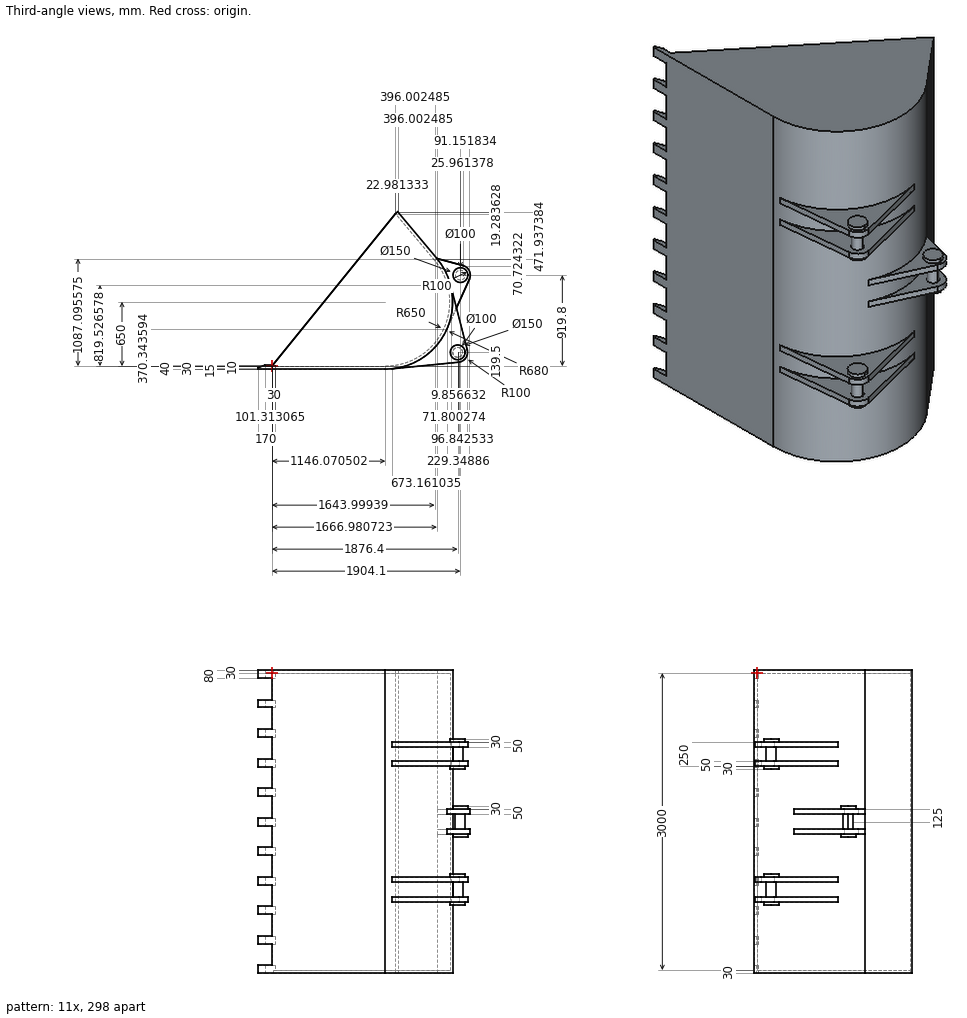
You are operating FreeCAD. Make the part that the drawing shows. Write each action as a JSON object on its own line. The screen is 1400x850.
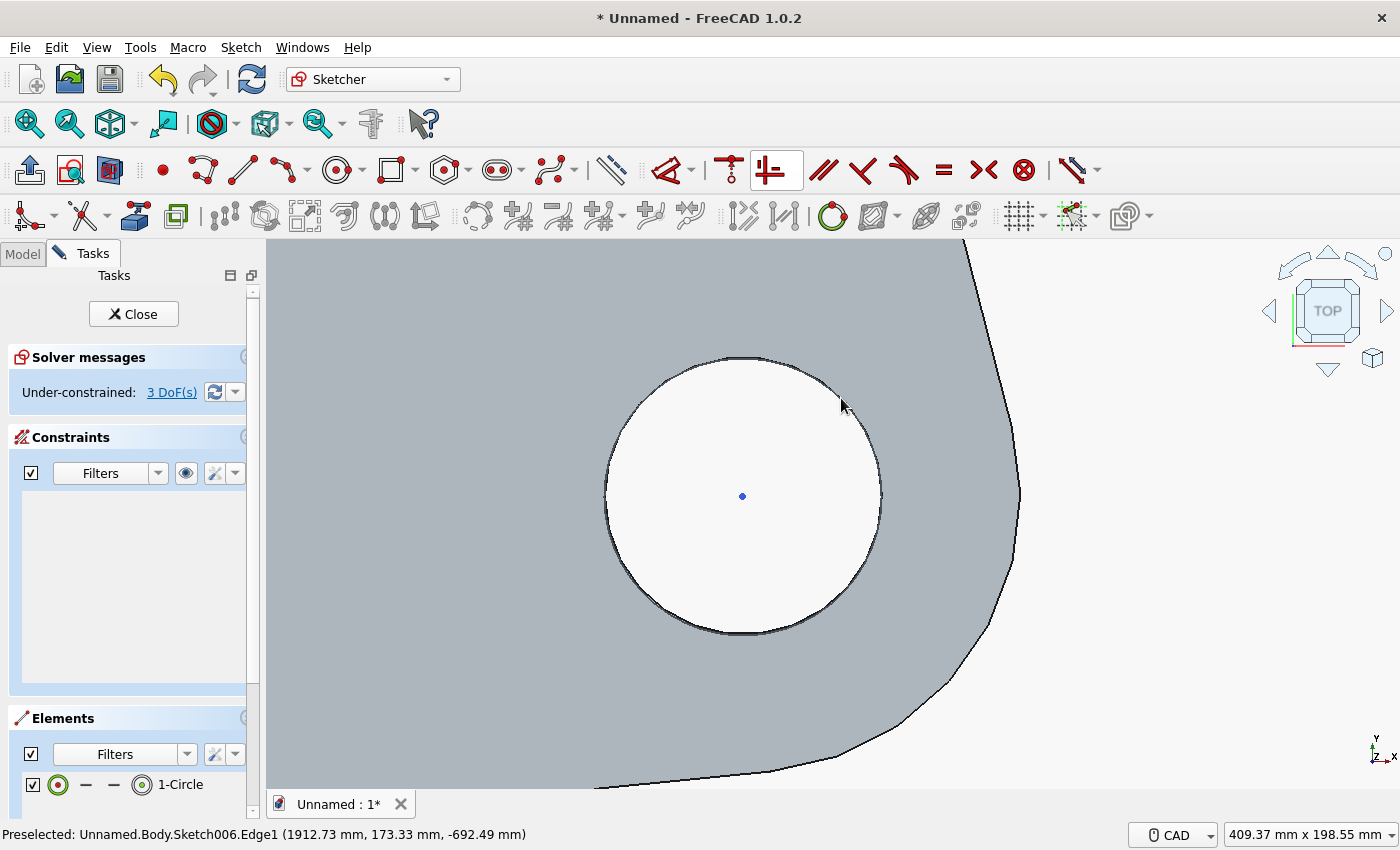
{"action": "left_click", "coordinate": [666, 170]}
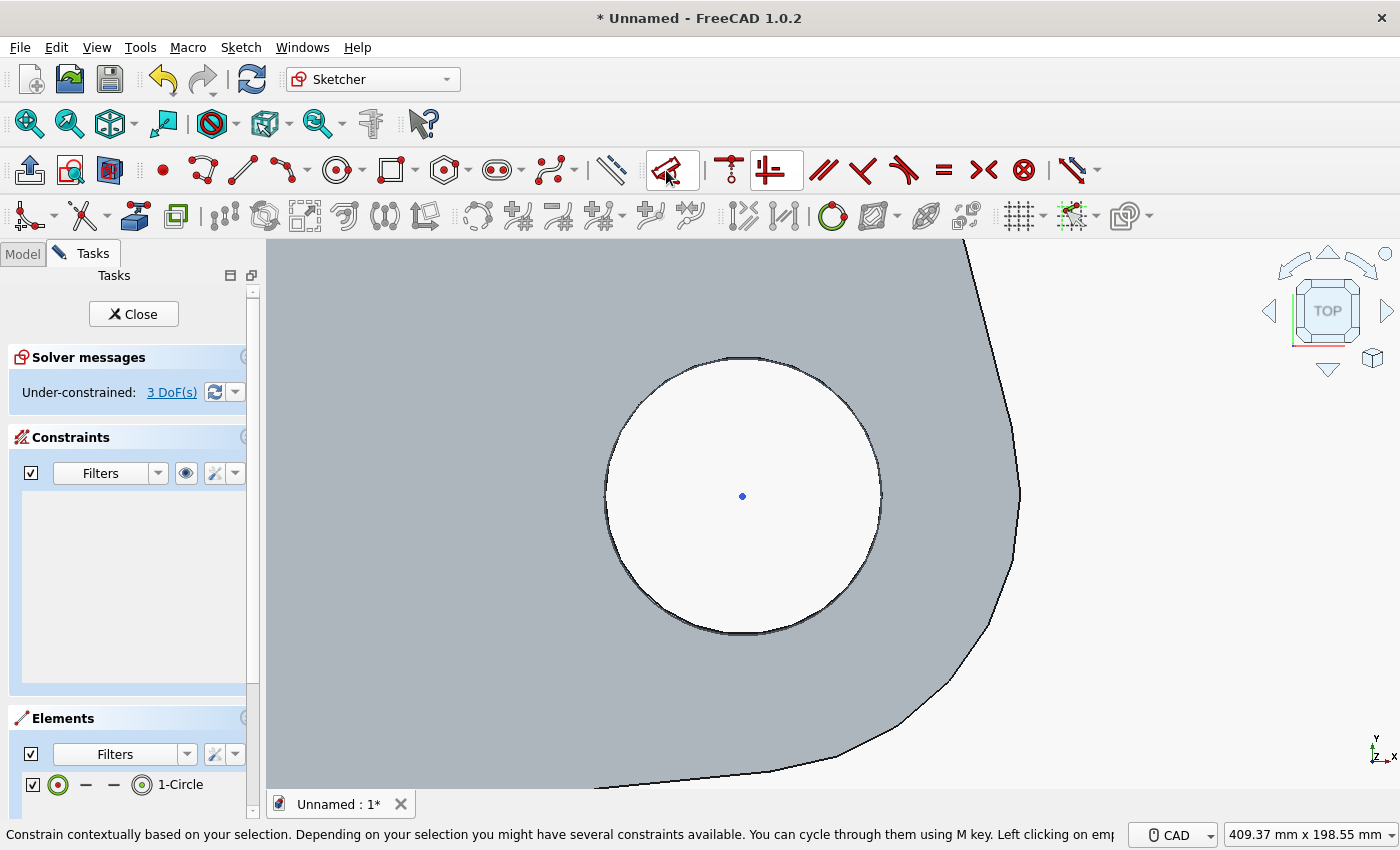
{"action": "left_click", "coordinate": [841, 399]}
{"action": "left_click", "coordinate": [864, 376]}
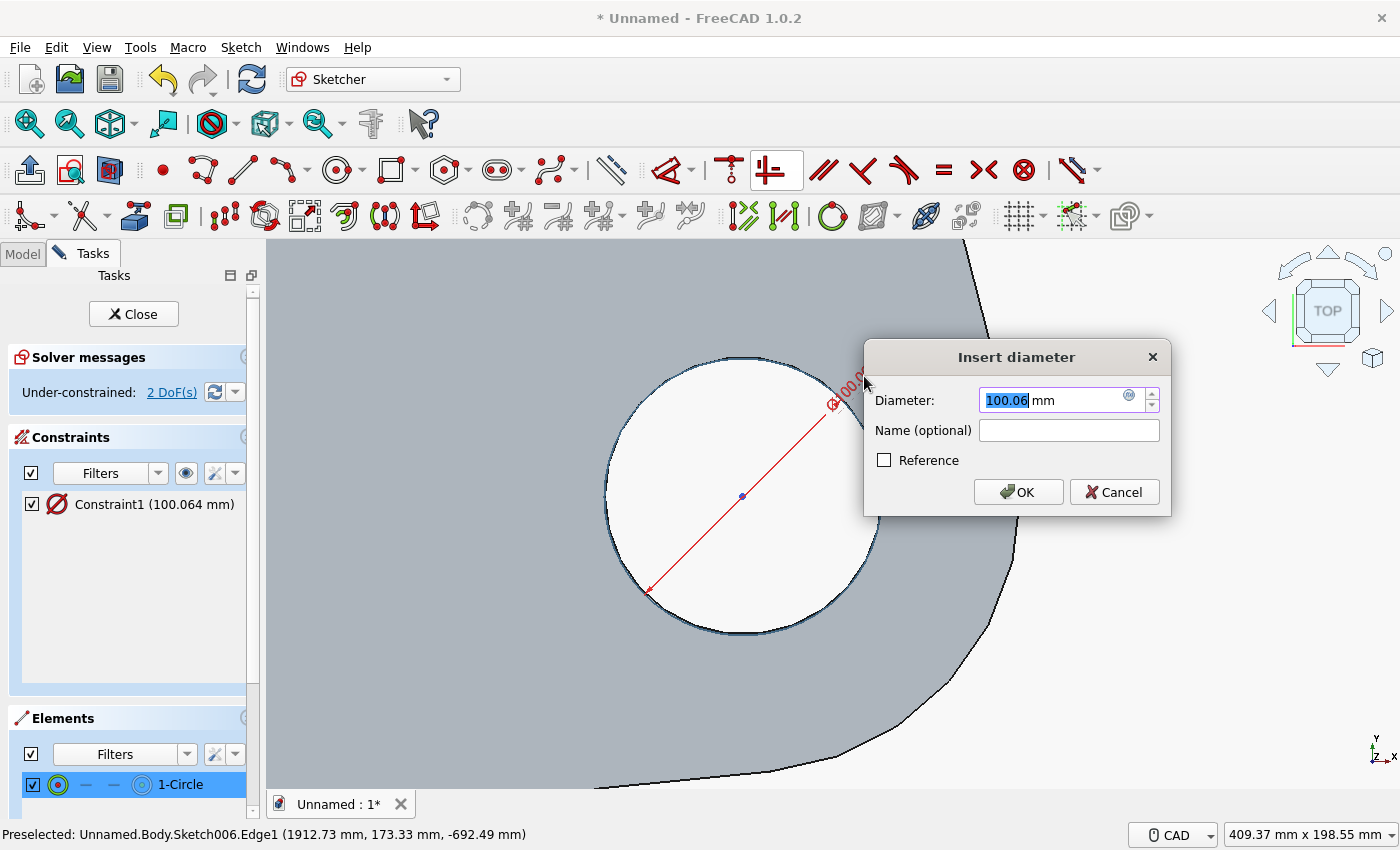
{"action": "type", "text": "100"}
{"action": "key", "text": "Return"}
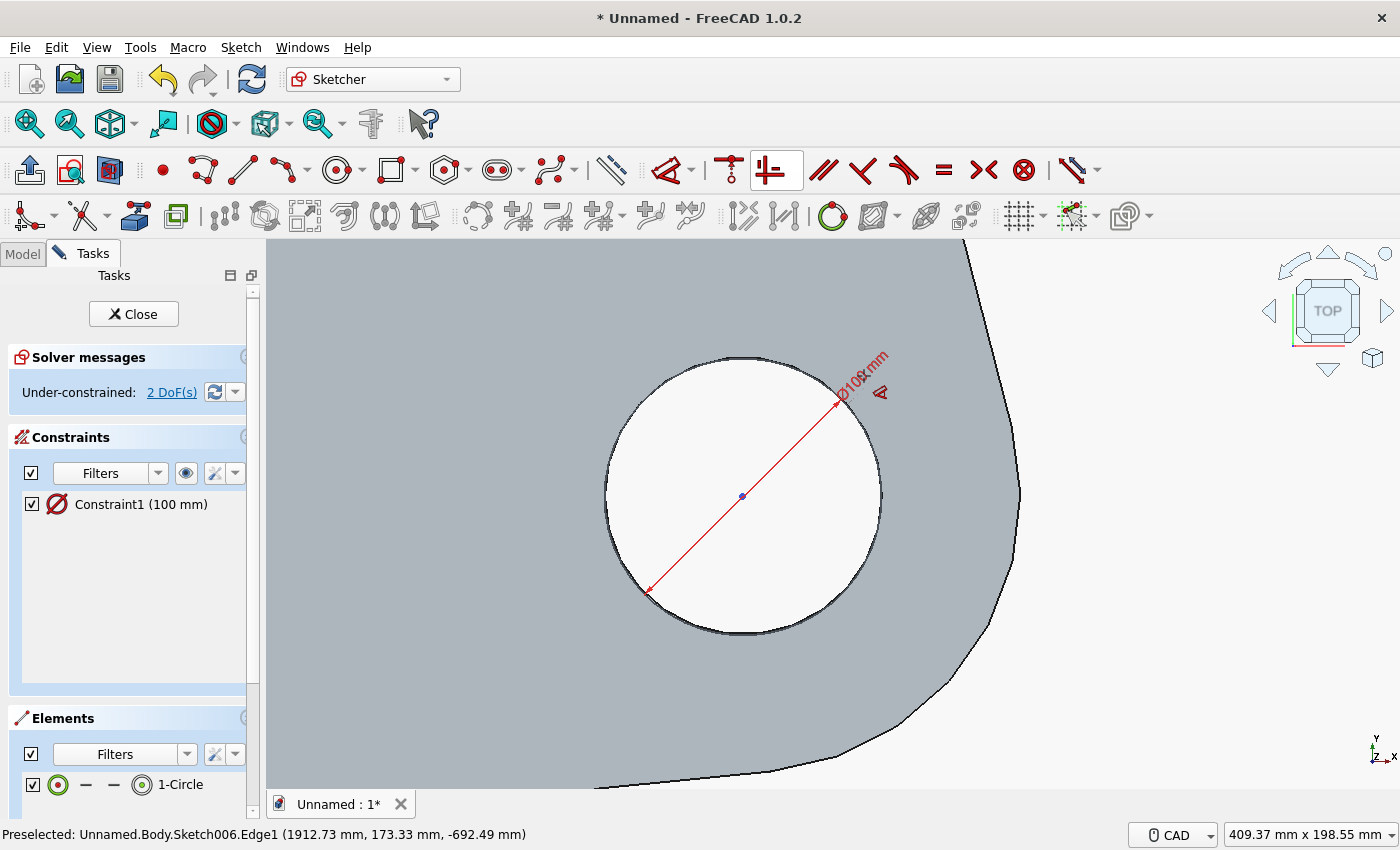
{"action": "left_click", "coordinate": [743, 497]}
{"action": "left_click", "coordinate": [777, 568]}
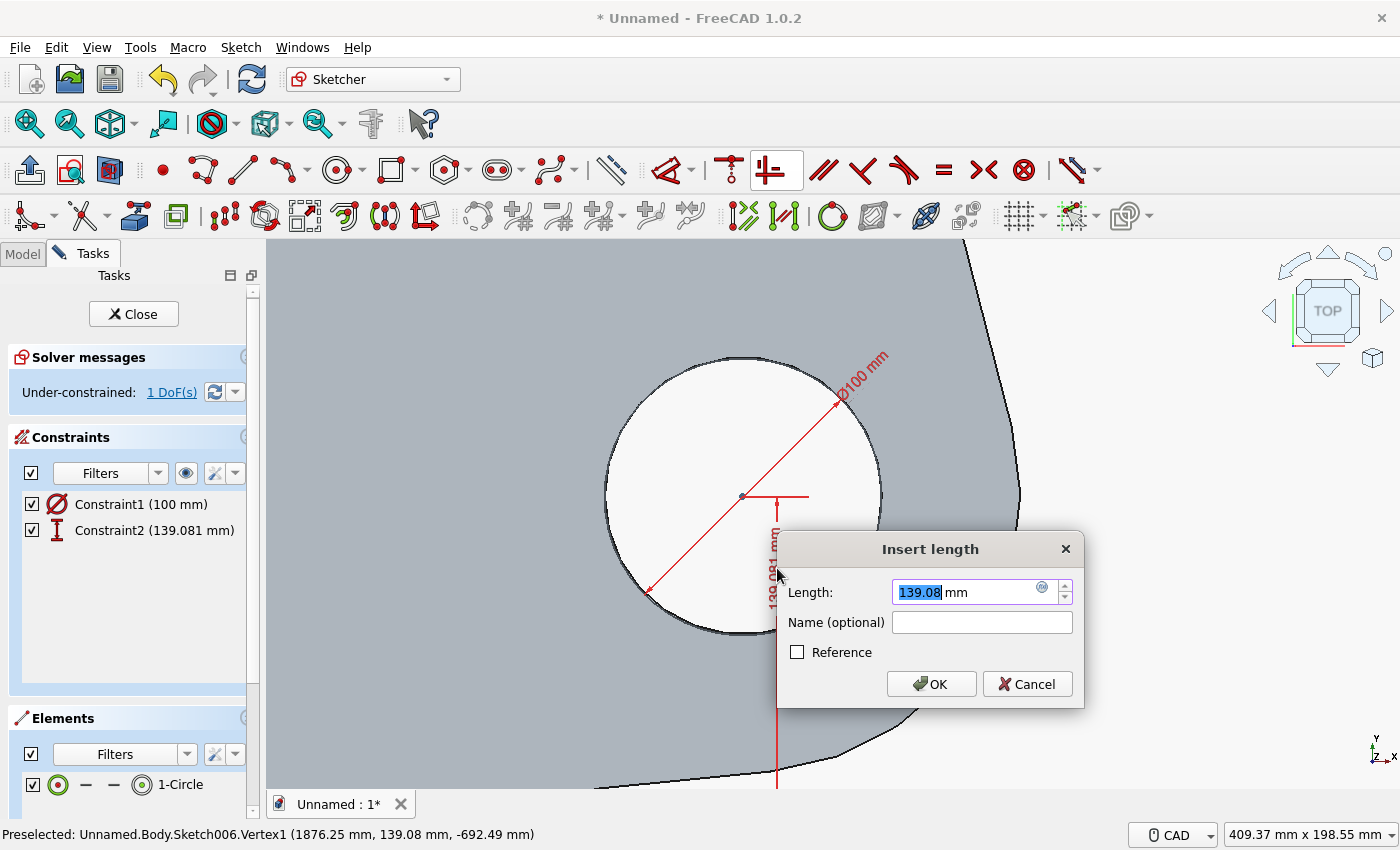
{"action": "type", "text": "139.5"}
{"action": "key", "text": "Return"}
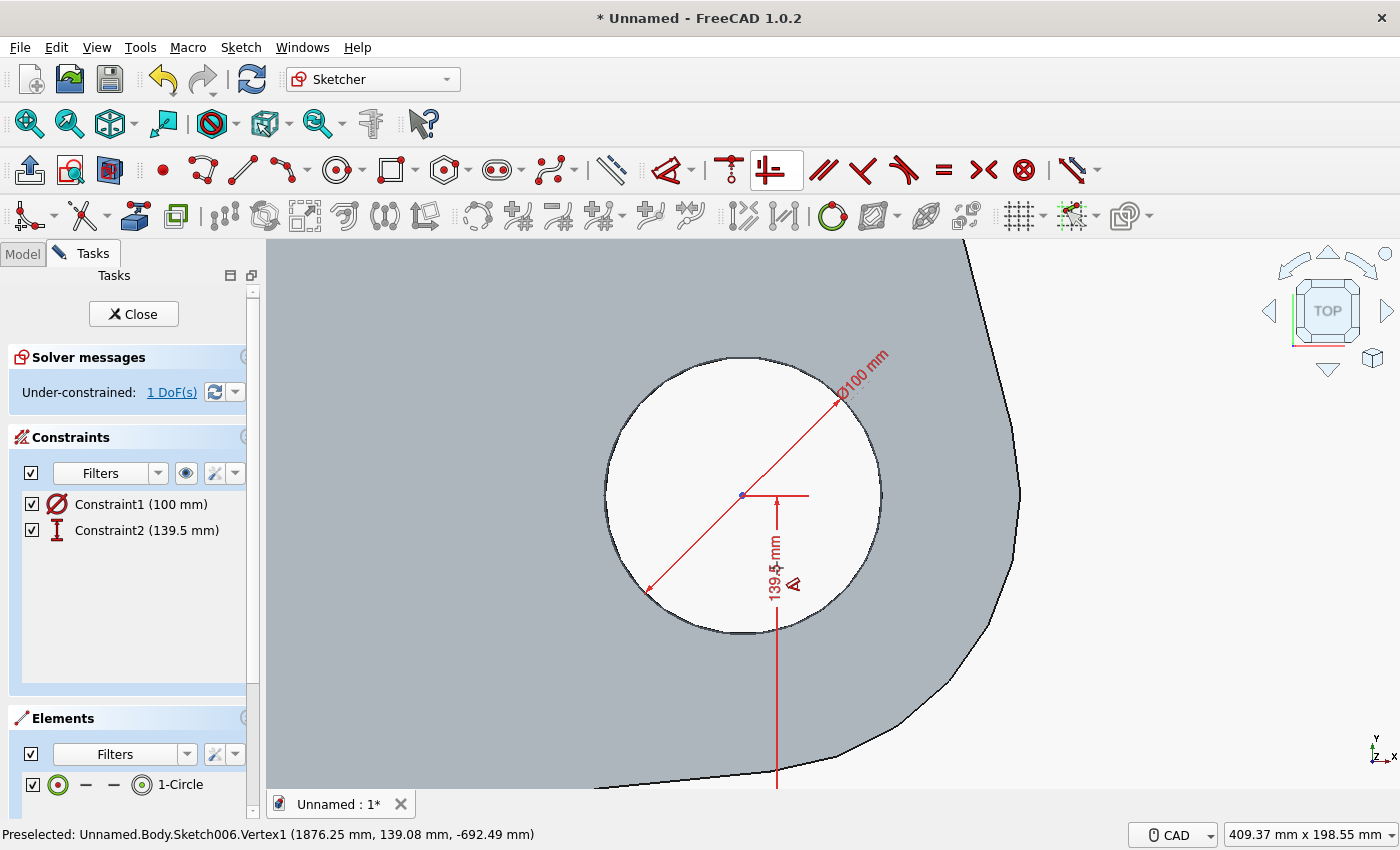
{"action": "left_click", "coordinate": [743, 496]}
{"action": "left_click", "coordinate": [519, 462]}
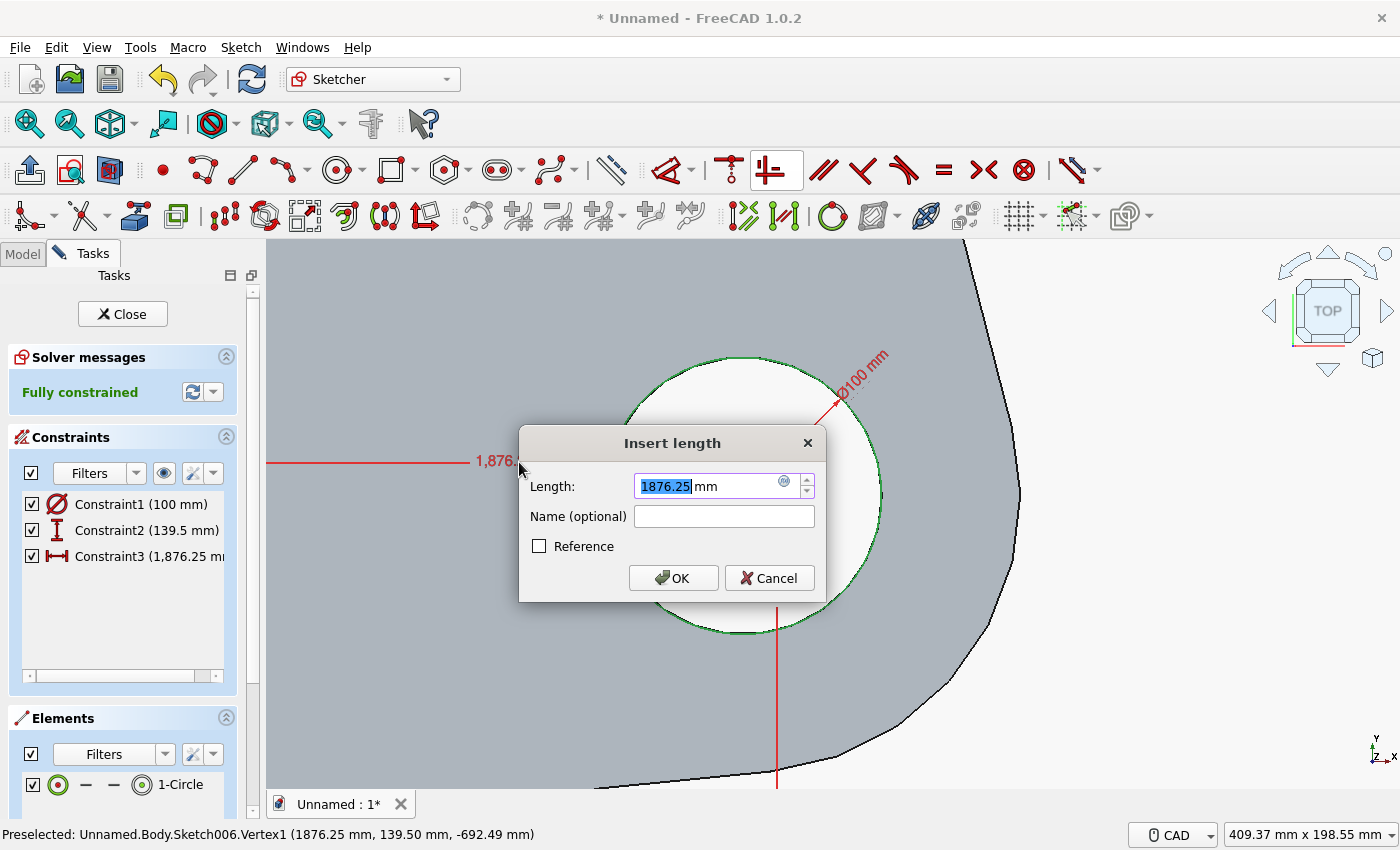
{"action": "type", "text": "1876.4"}
{"action": "key", "text": "Return"}
{"action": "key", "text": "Escape"}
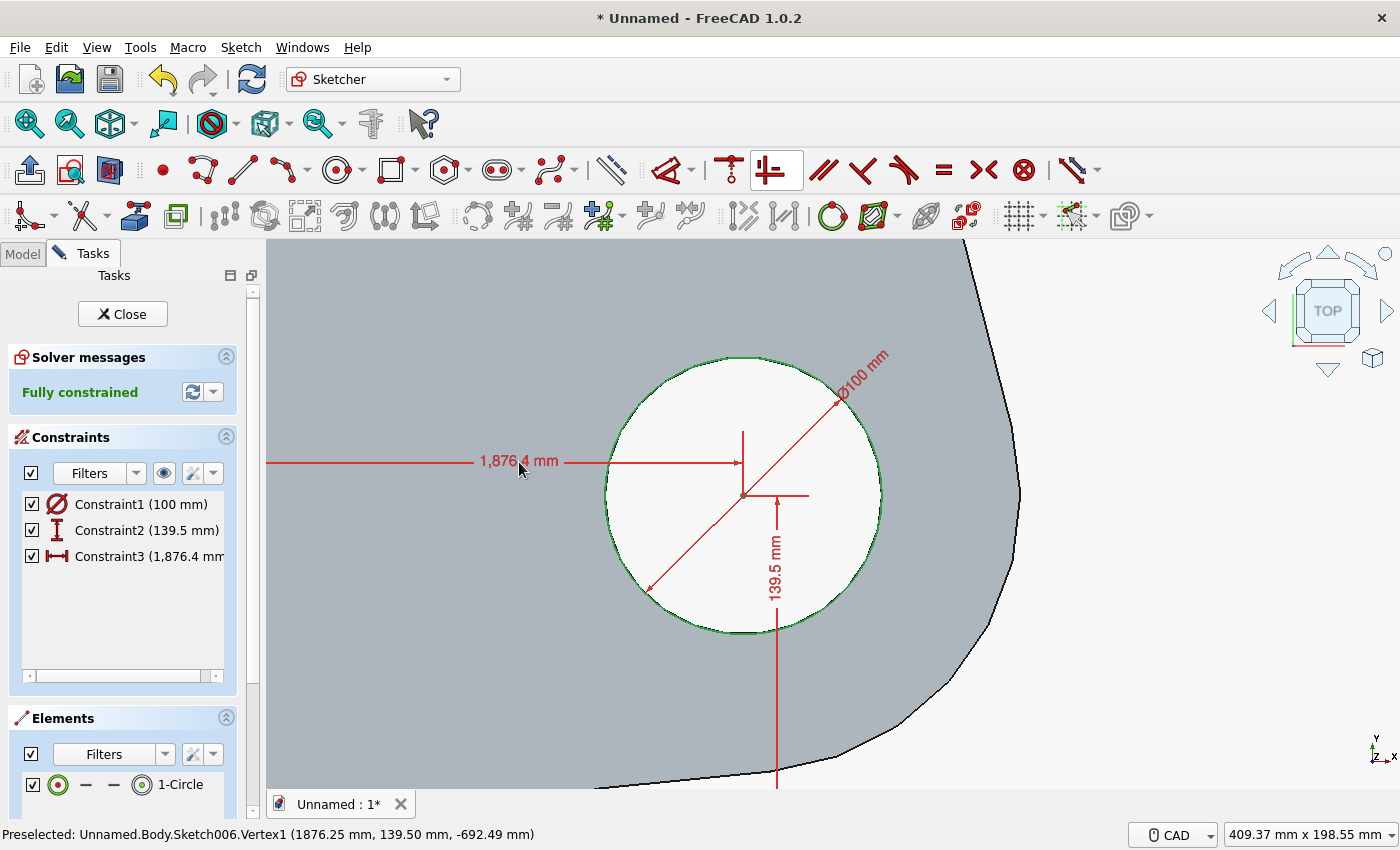
{"action": "left_click", "coordinate": [123, 314]}